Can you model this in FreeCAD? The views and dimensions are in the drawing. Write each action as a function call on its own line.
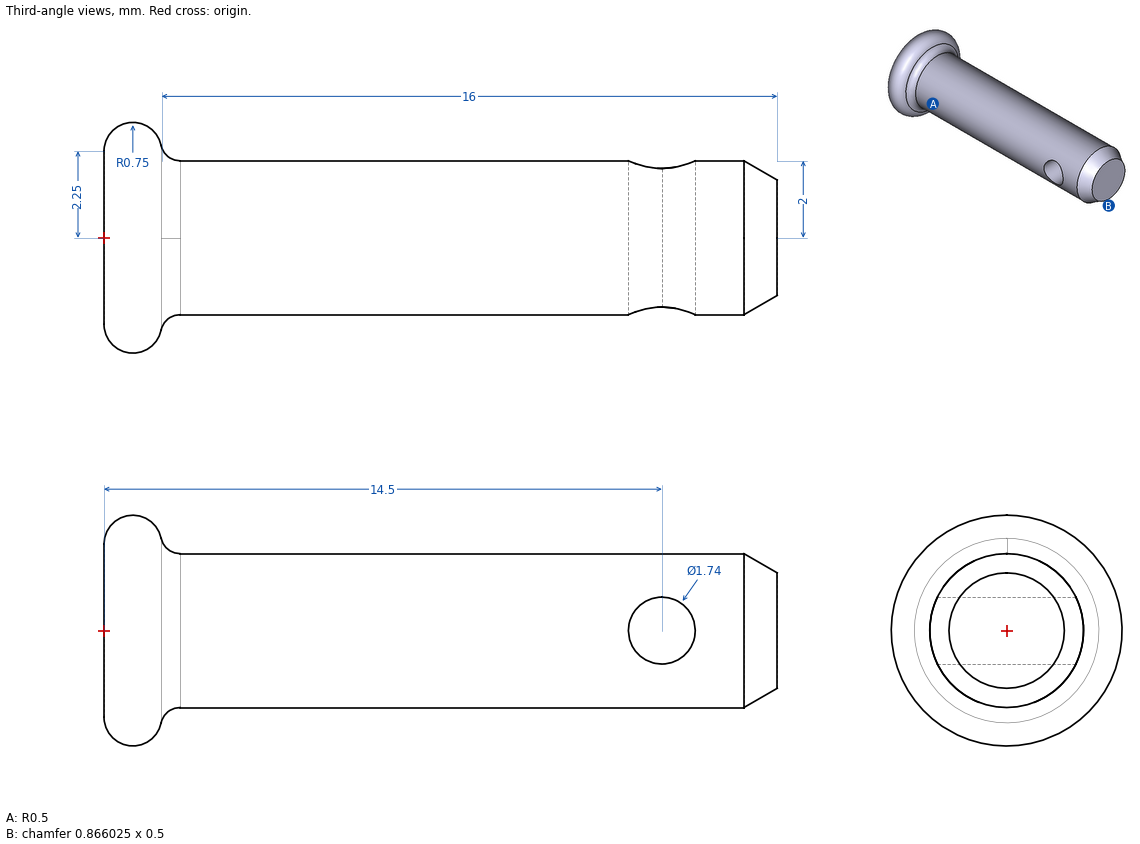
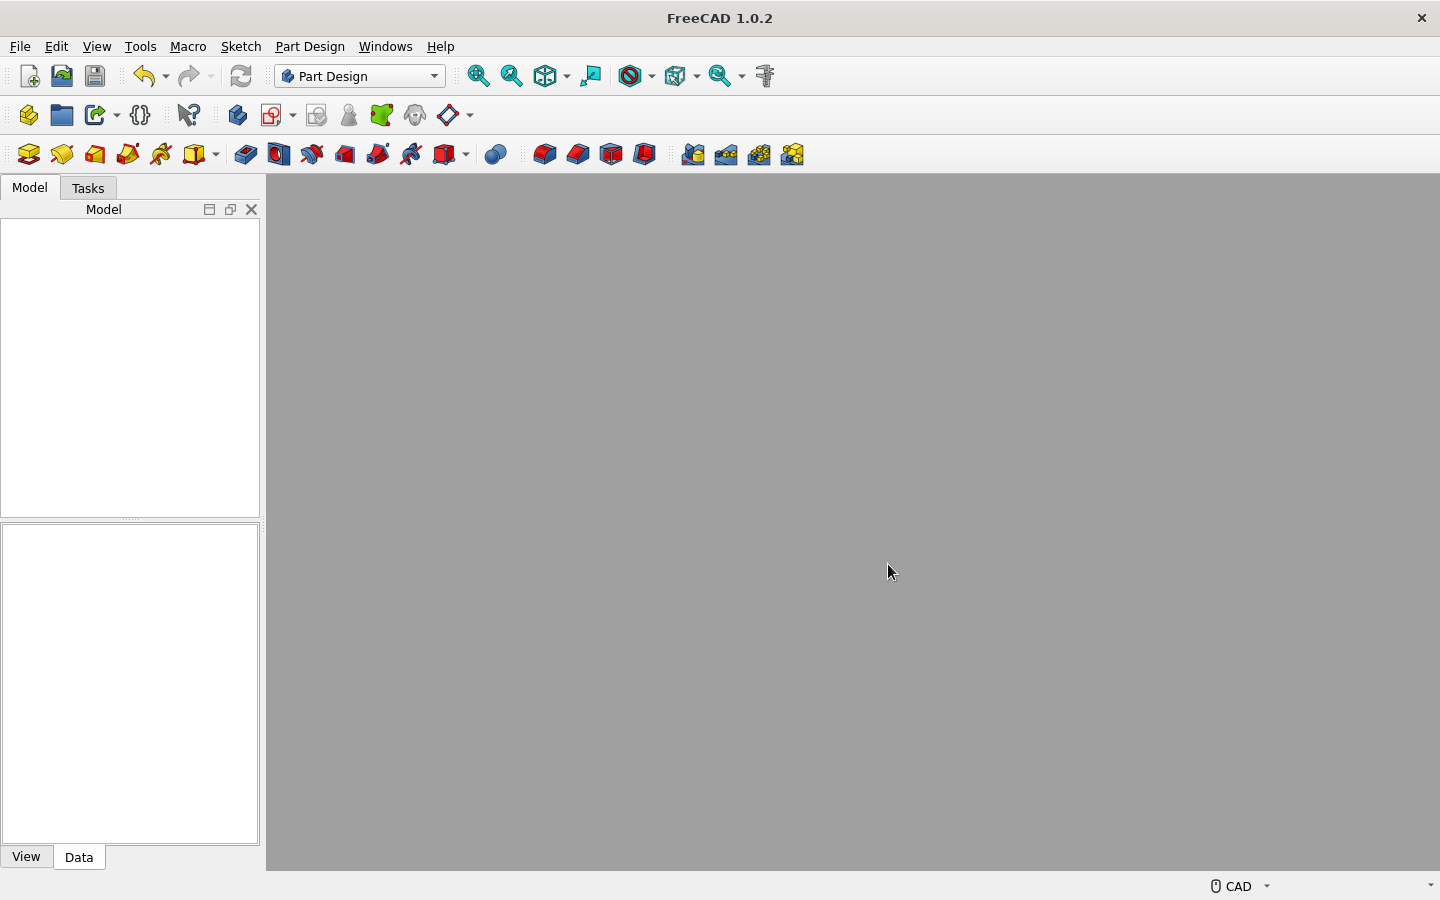
click(29, 76)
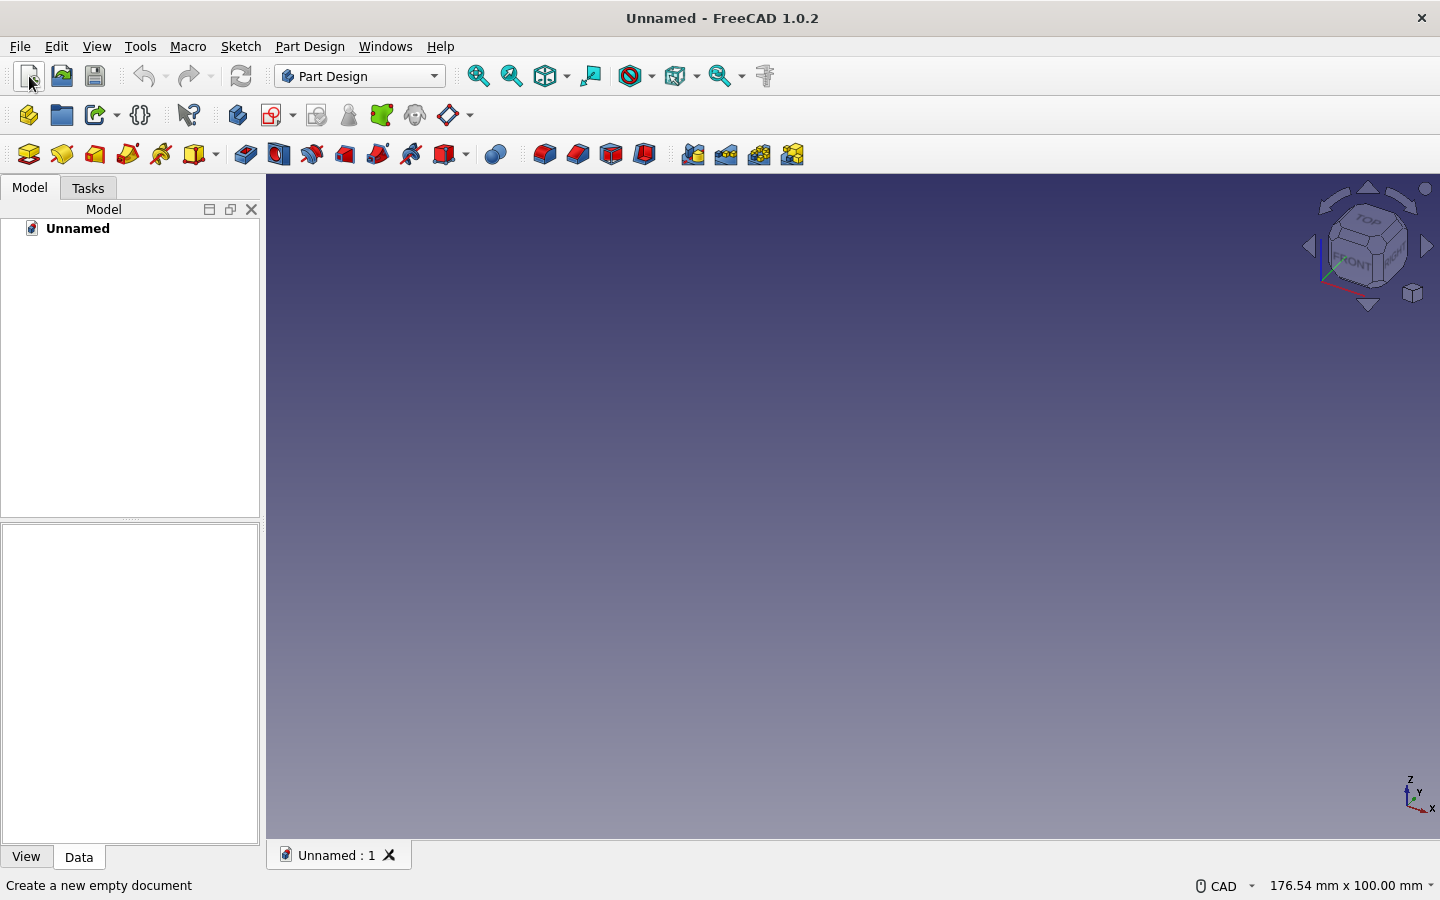
click(270, 116)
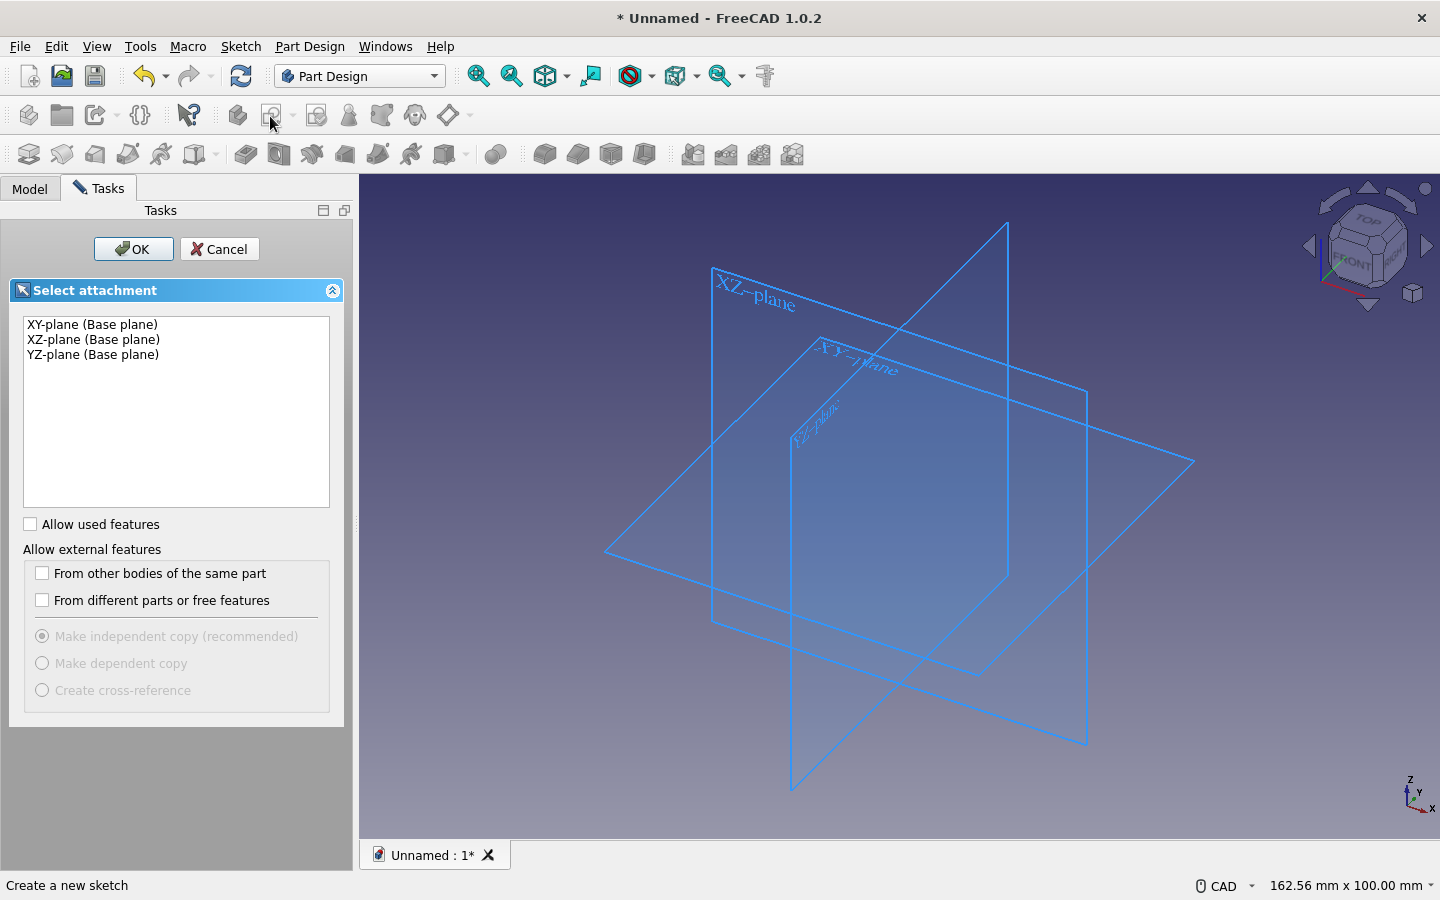
click(84, 324)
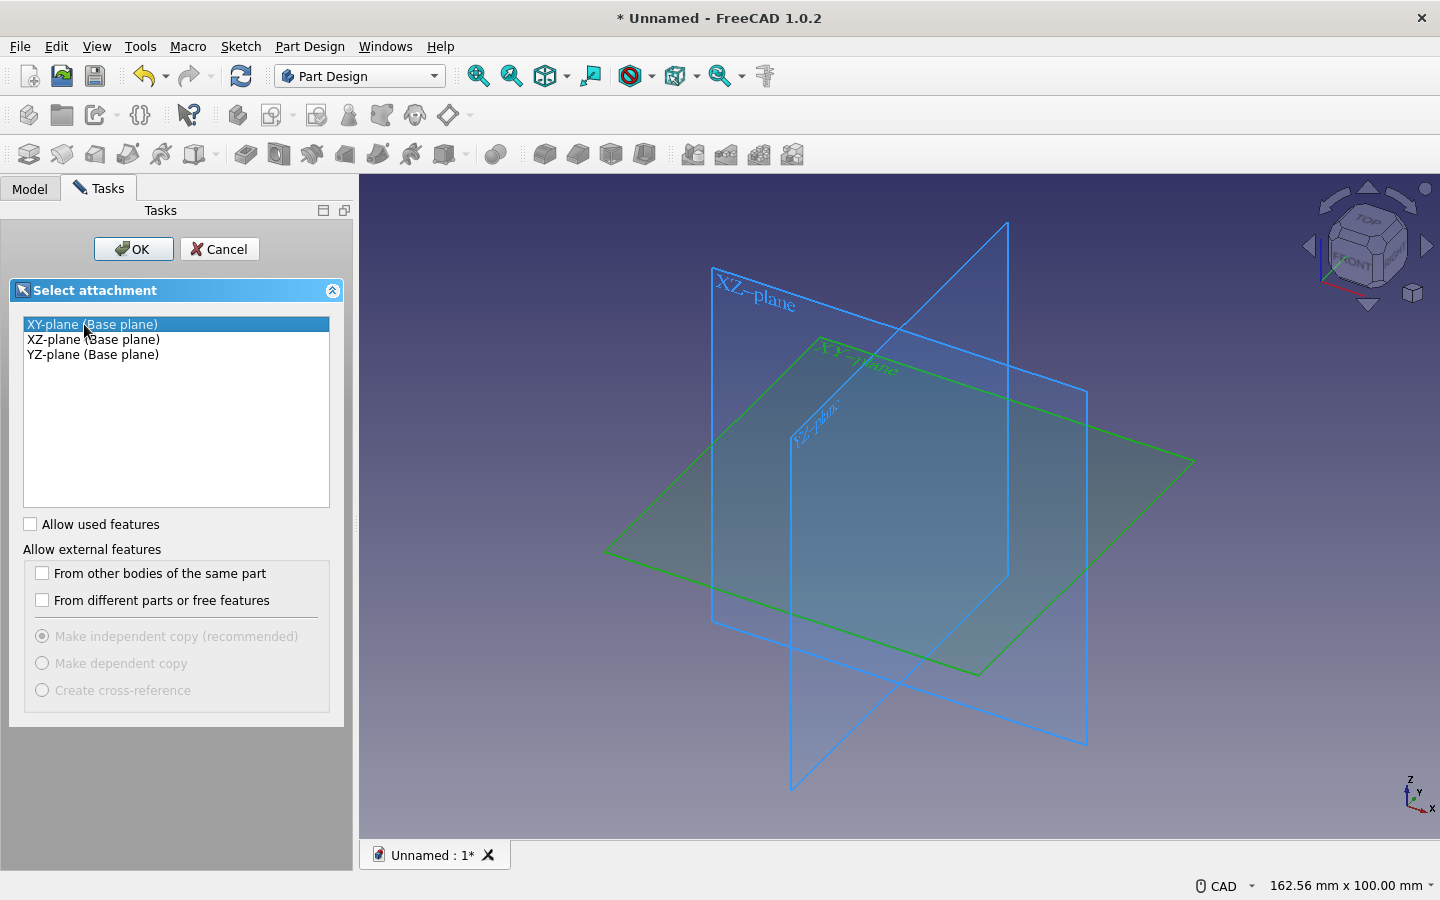
click(134, 249)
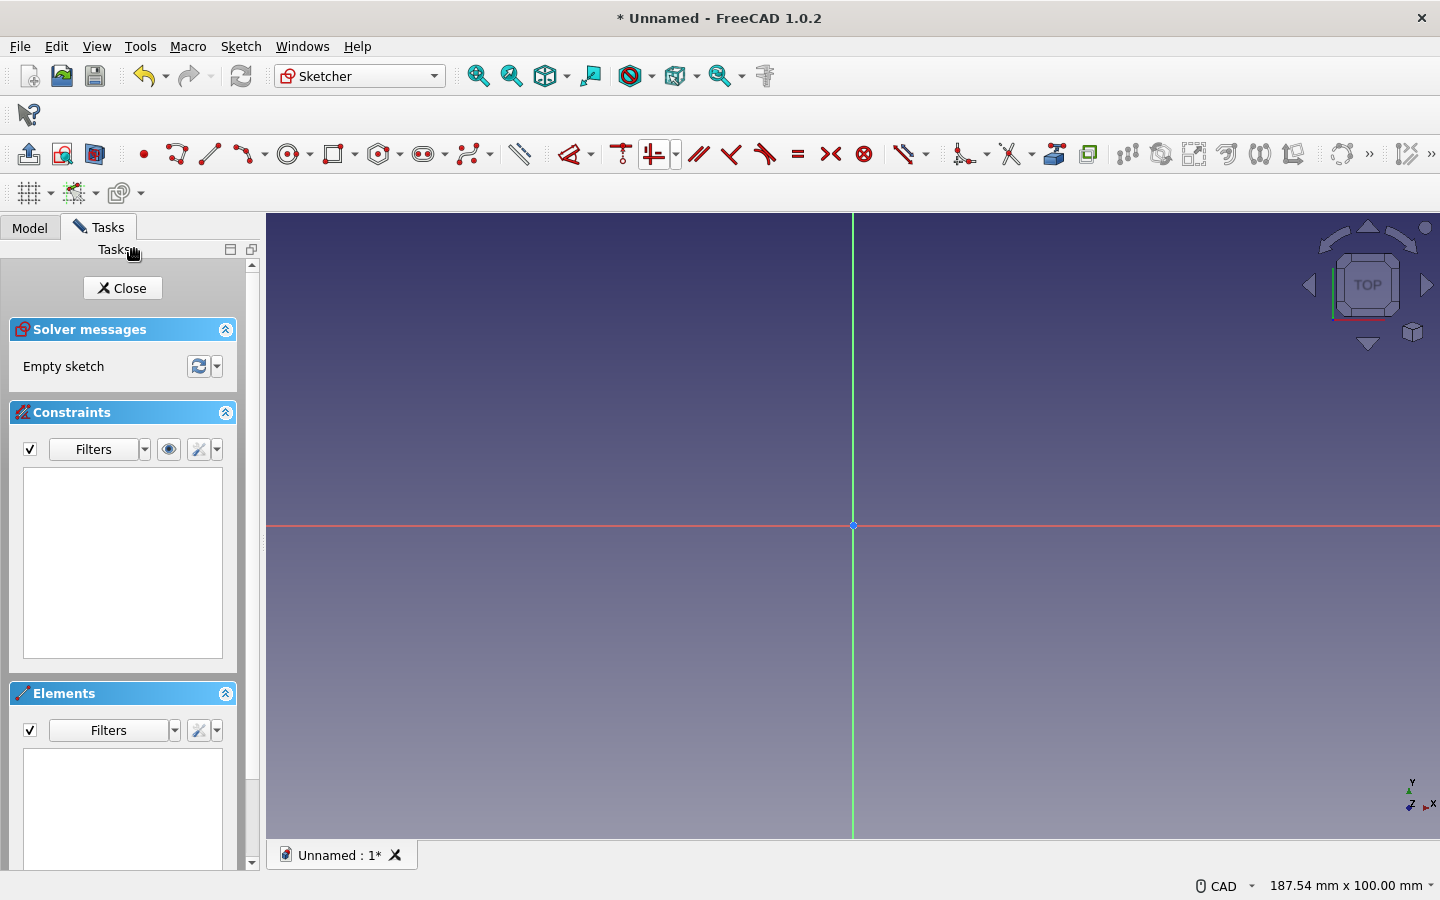
scroll(932, 515, up, 9)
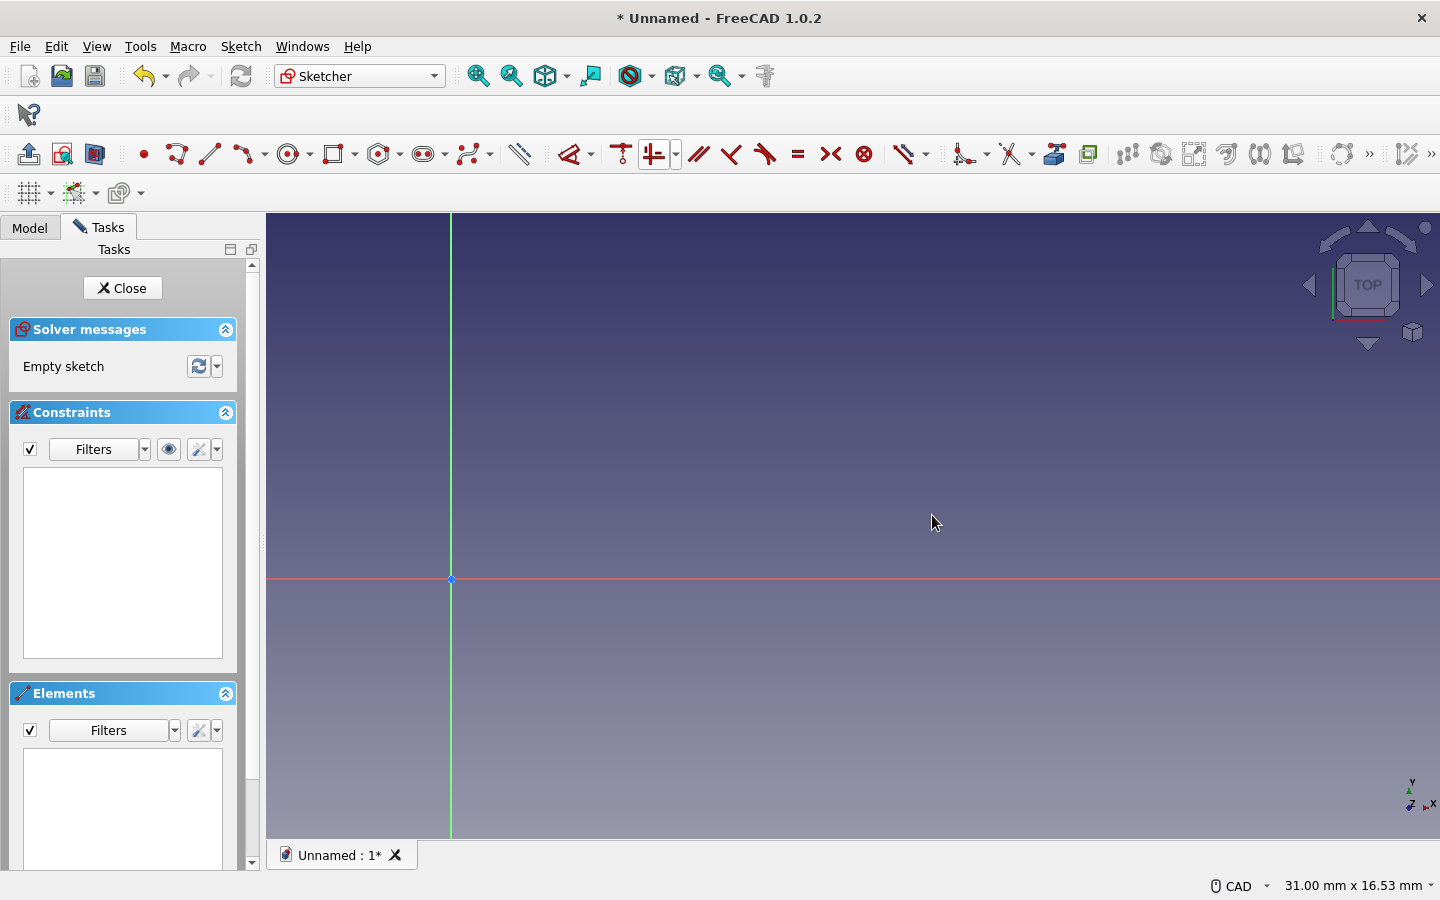
click(177, 154)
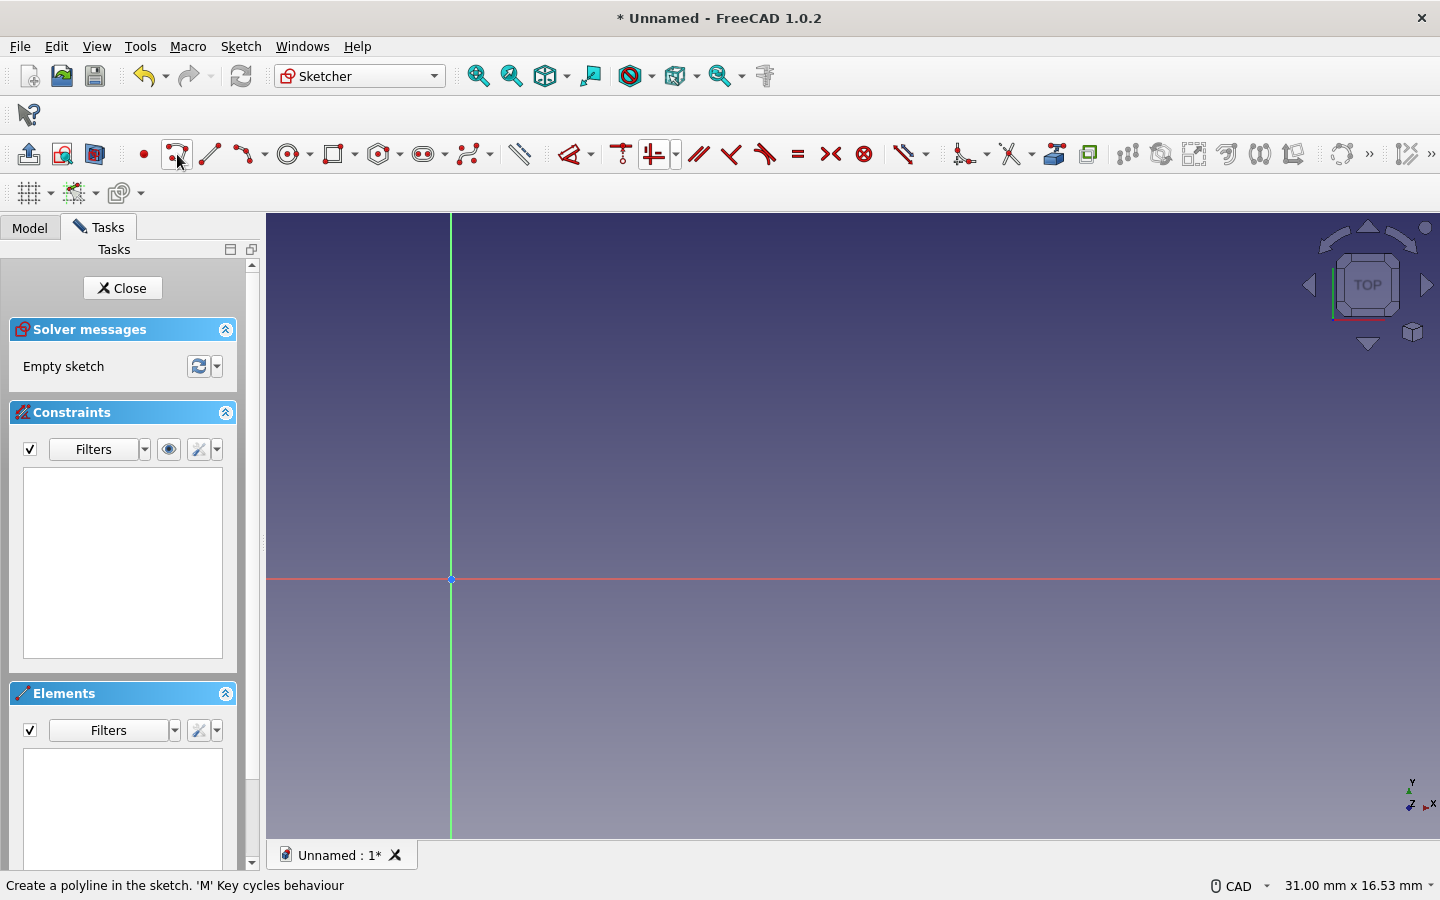
click(451, 494)
click(451, 579)
click(1114, 570)
click(1114, 503)
click(508, 503)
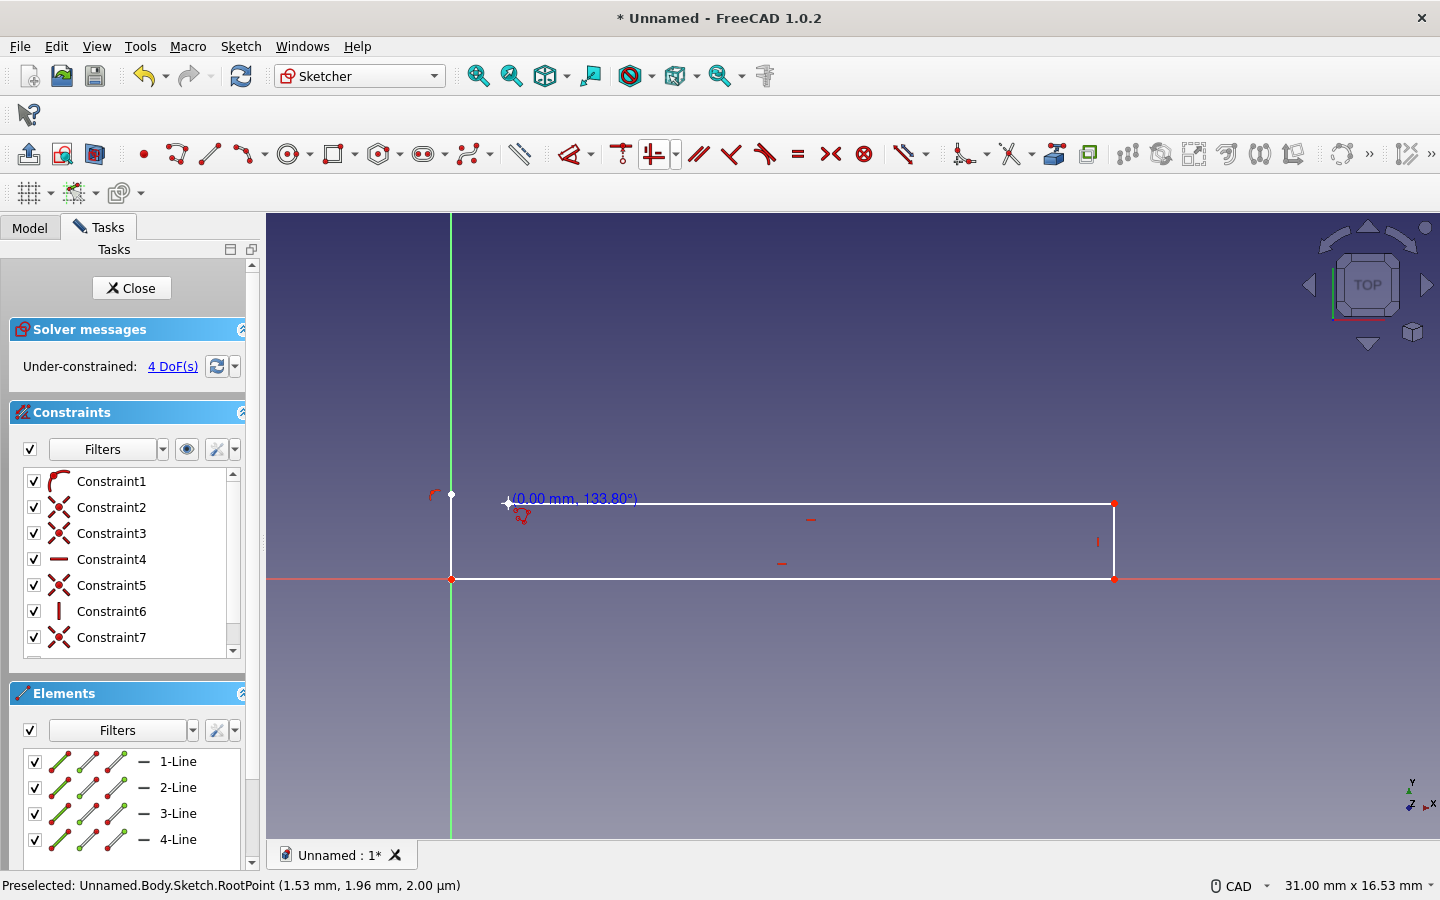
scroll(508, 494, up, 3)